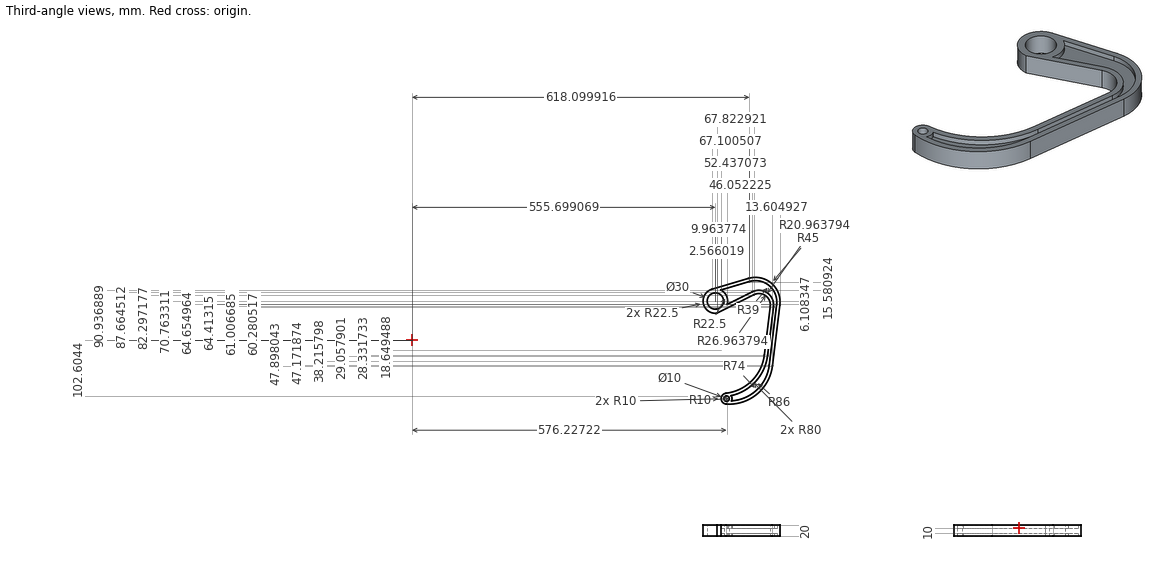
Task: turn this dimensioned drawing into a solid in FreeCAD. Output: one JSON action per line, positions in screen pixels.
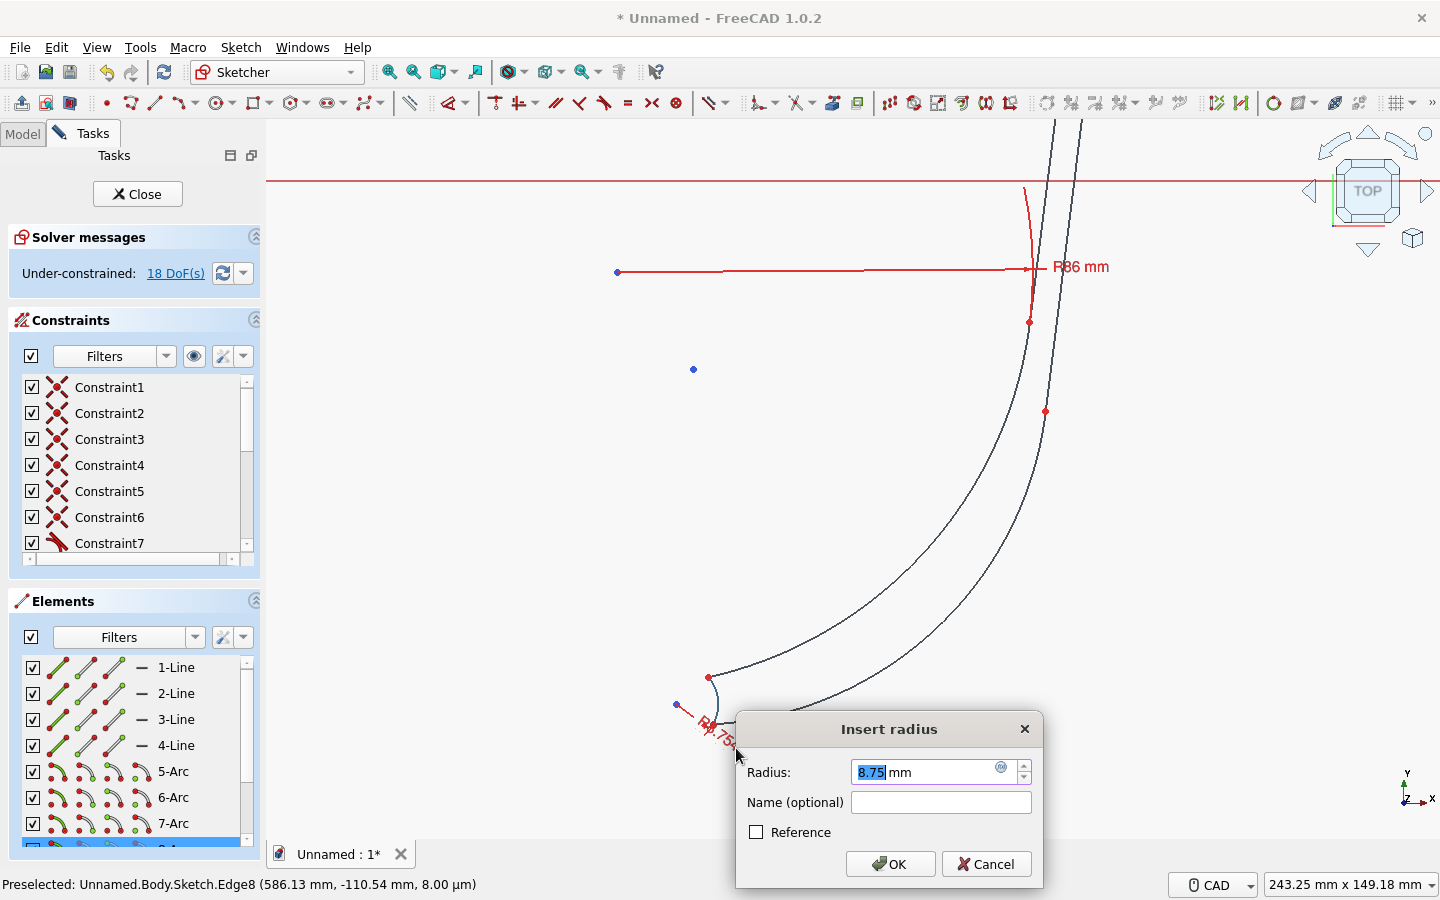
{"action": "type", "text": "10"}
{"action": "key", "text": "Return"}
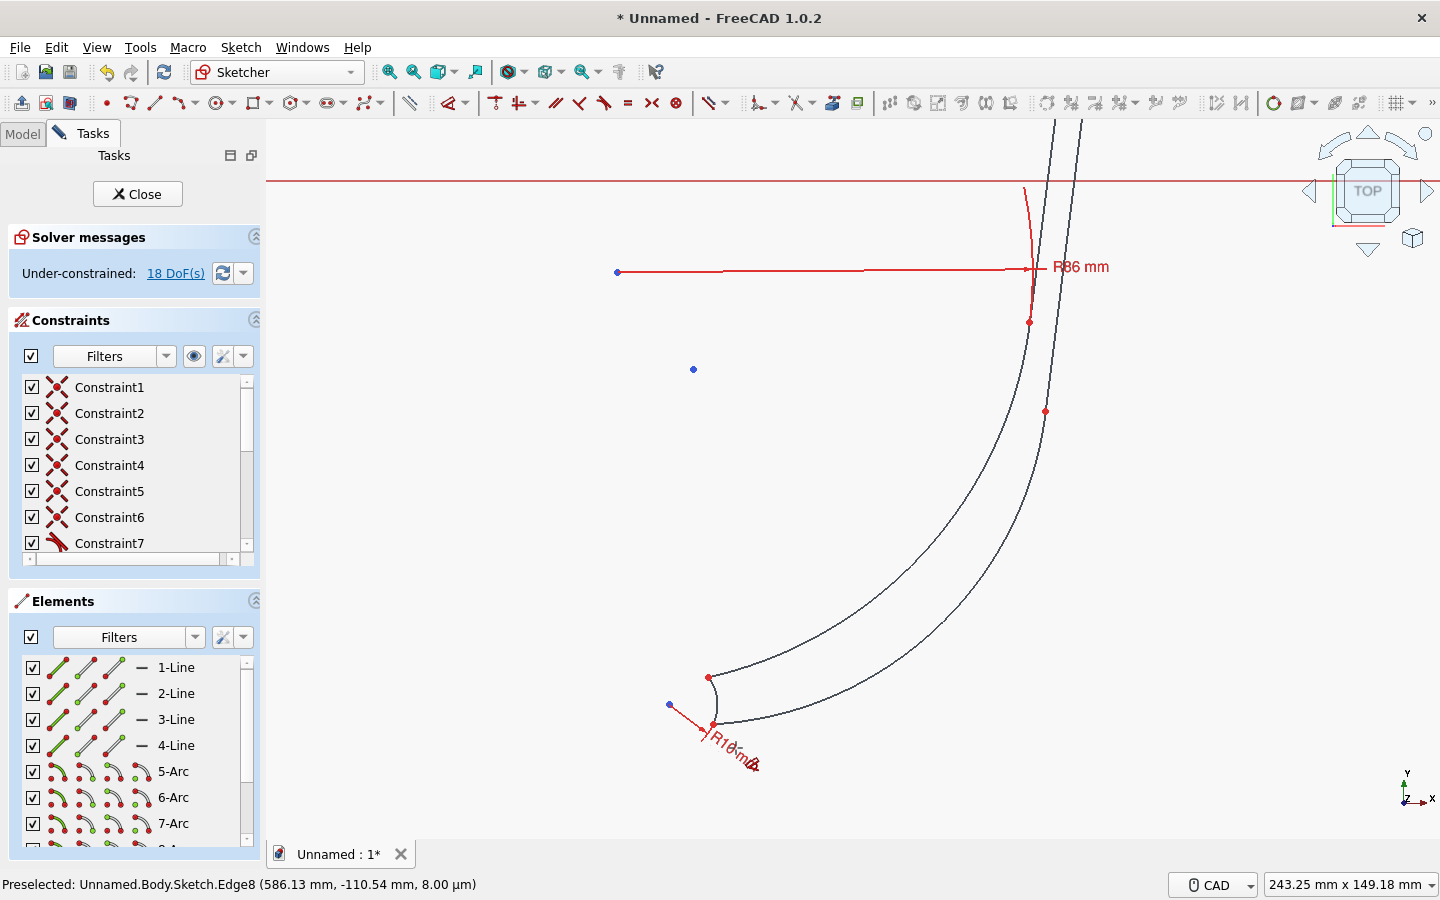
{"action": "left_click", "coordinate": [856, 685]}
{"action": "left_click", "coordinate": [871, 713]}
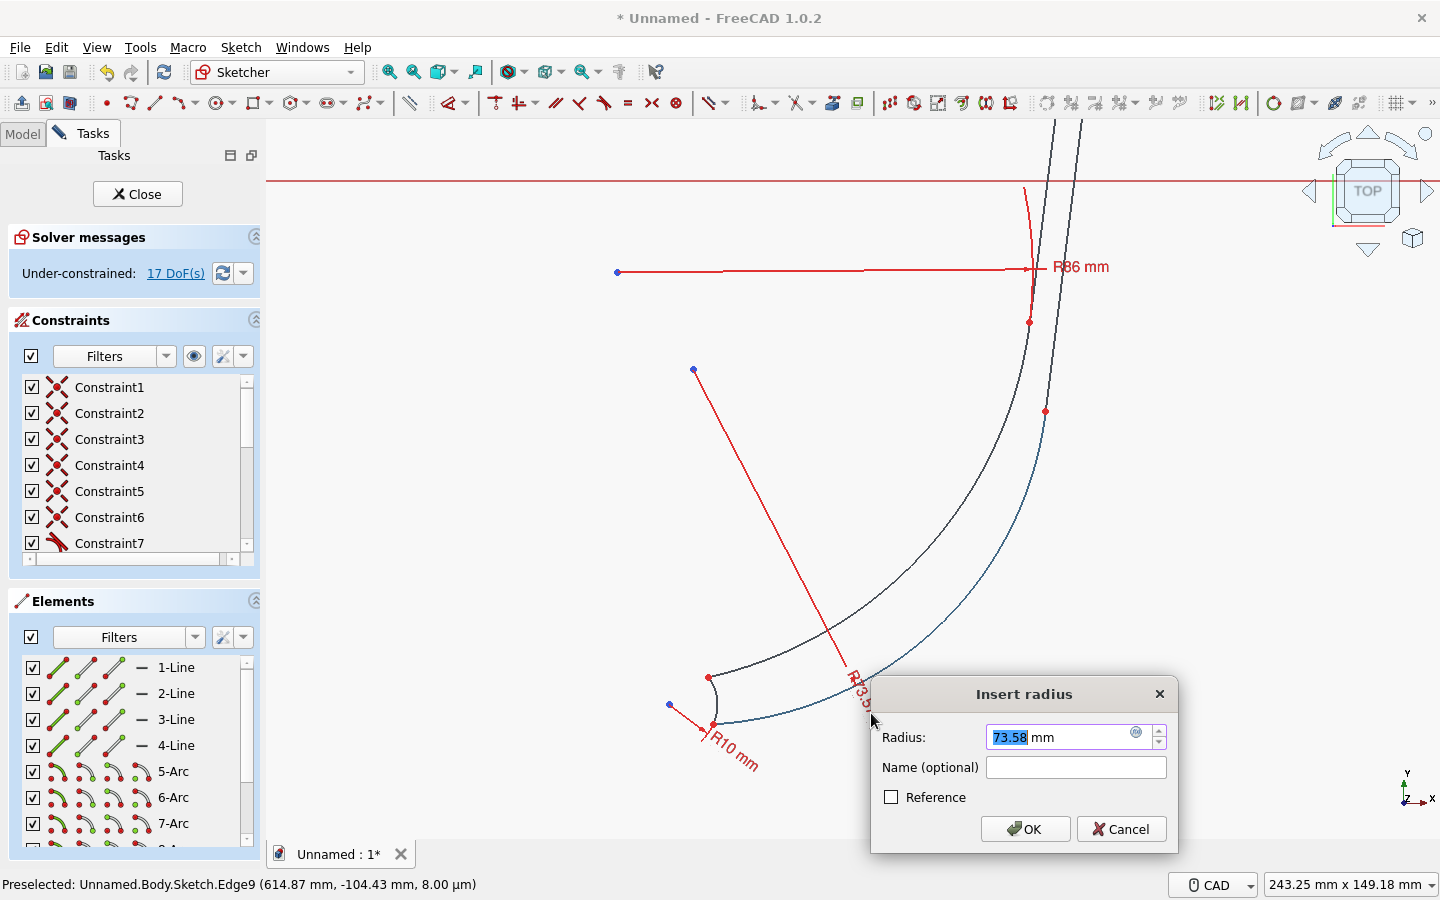
{"action": "type", "text": "74"}
{"action": "key", "text": "Return"}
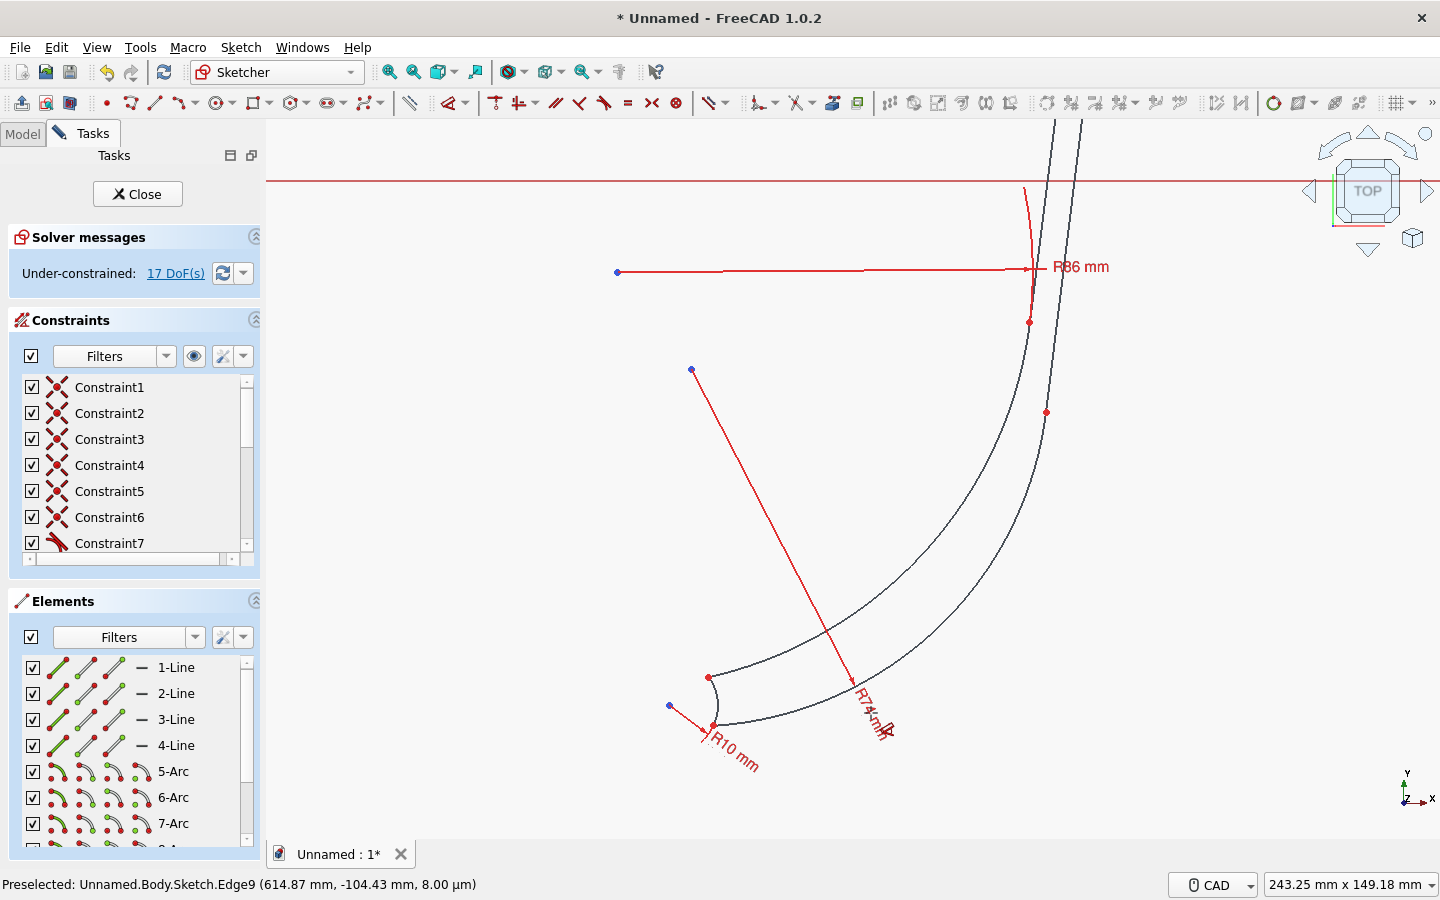
{"action": "scroll", "coordinate": [719, 711], "scroll_direction": "down", "scroll_amount": 4}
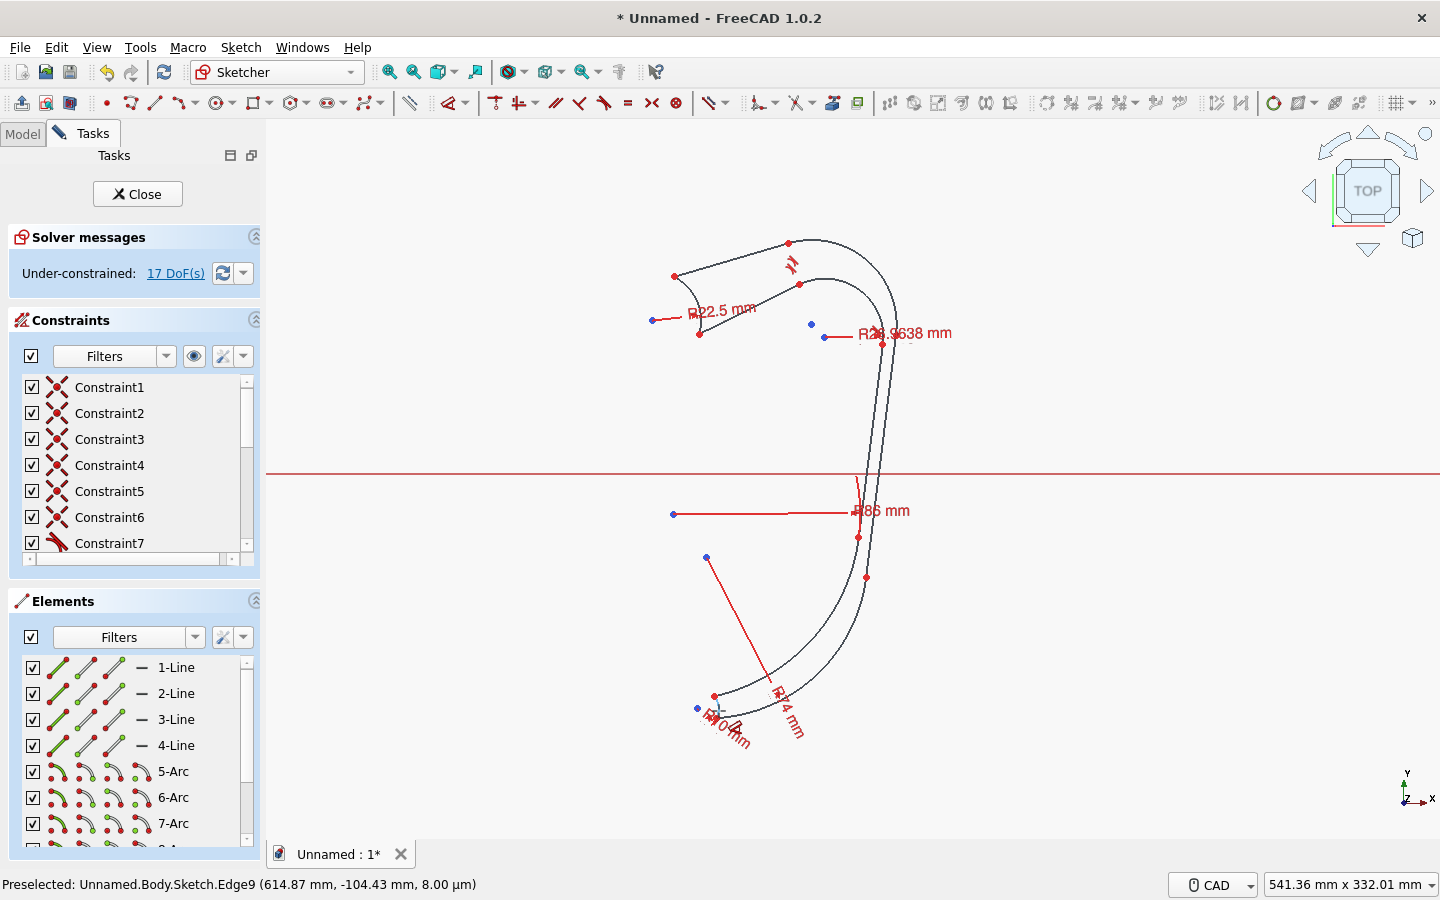
{"action": "left_click", "coordinate": [887, 286]}
{"action": "left_click", "coordinate": [915, 271]}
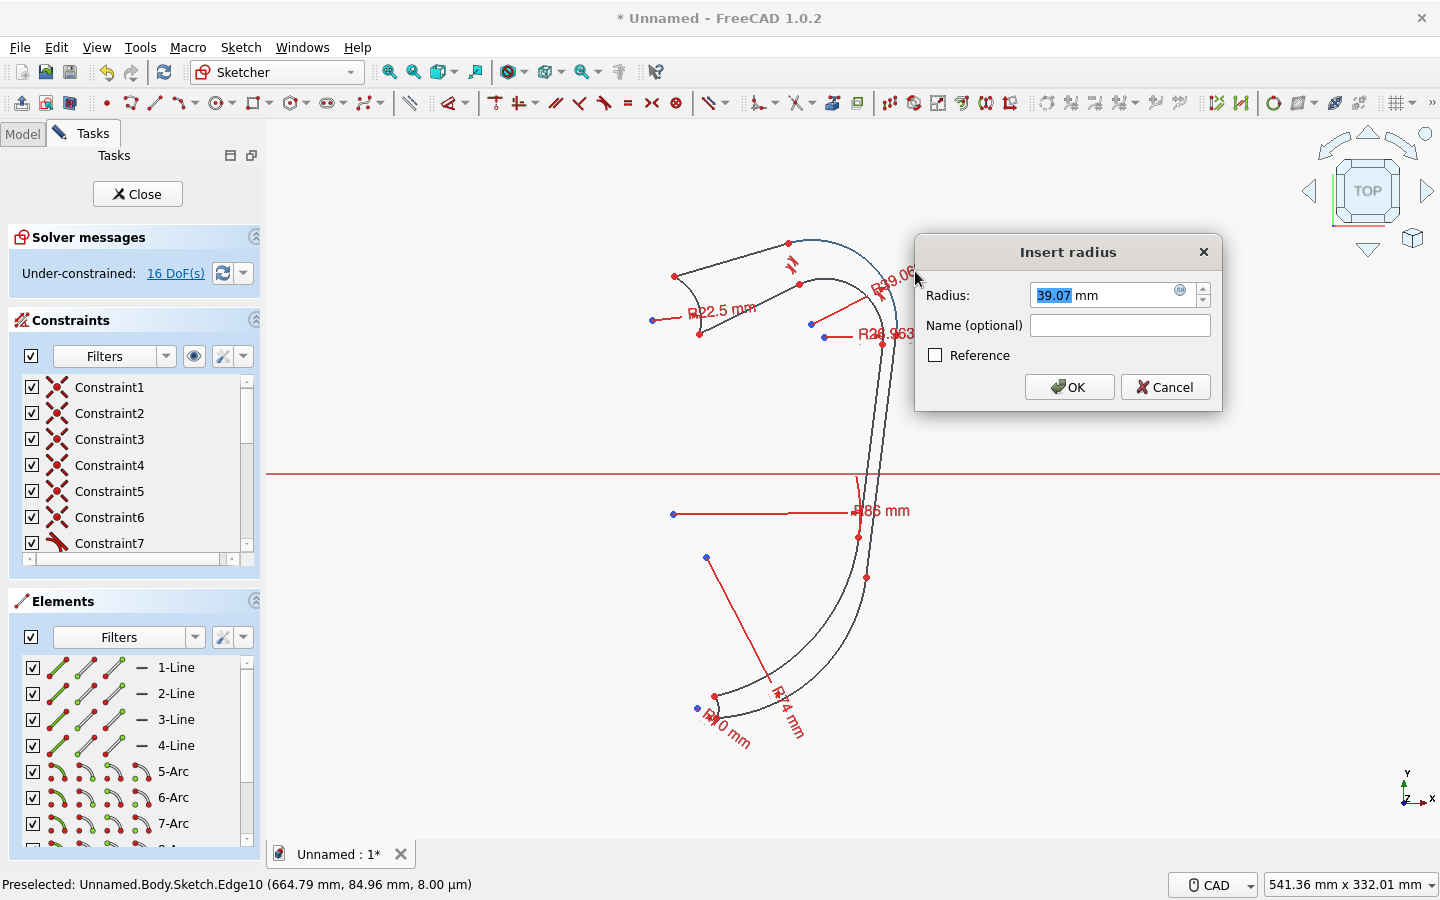
{"action": "type", "text": "39"}
{"action": "key", "text": "Return"}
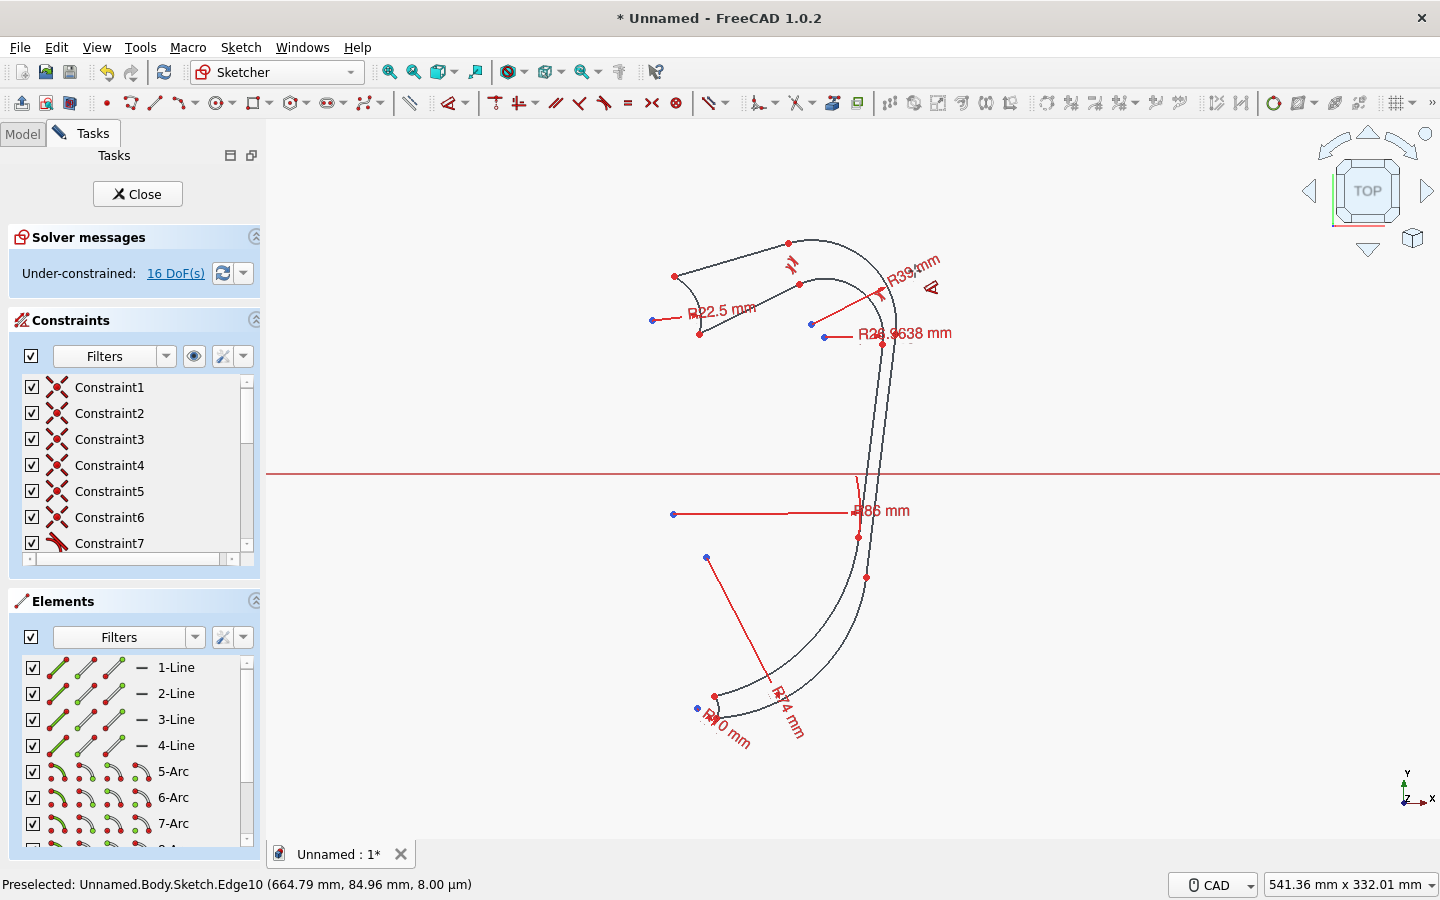
{"action": "left_click", "coordinate": [896, 335]}
{"action": "left_click", "coordinate": [930, 404]}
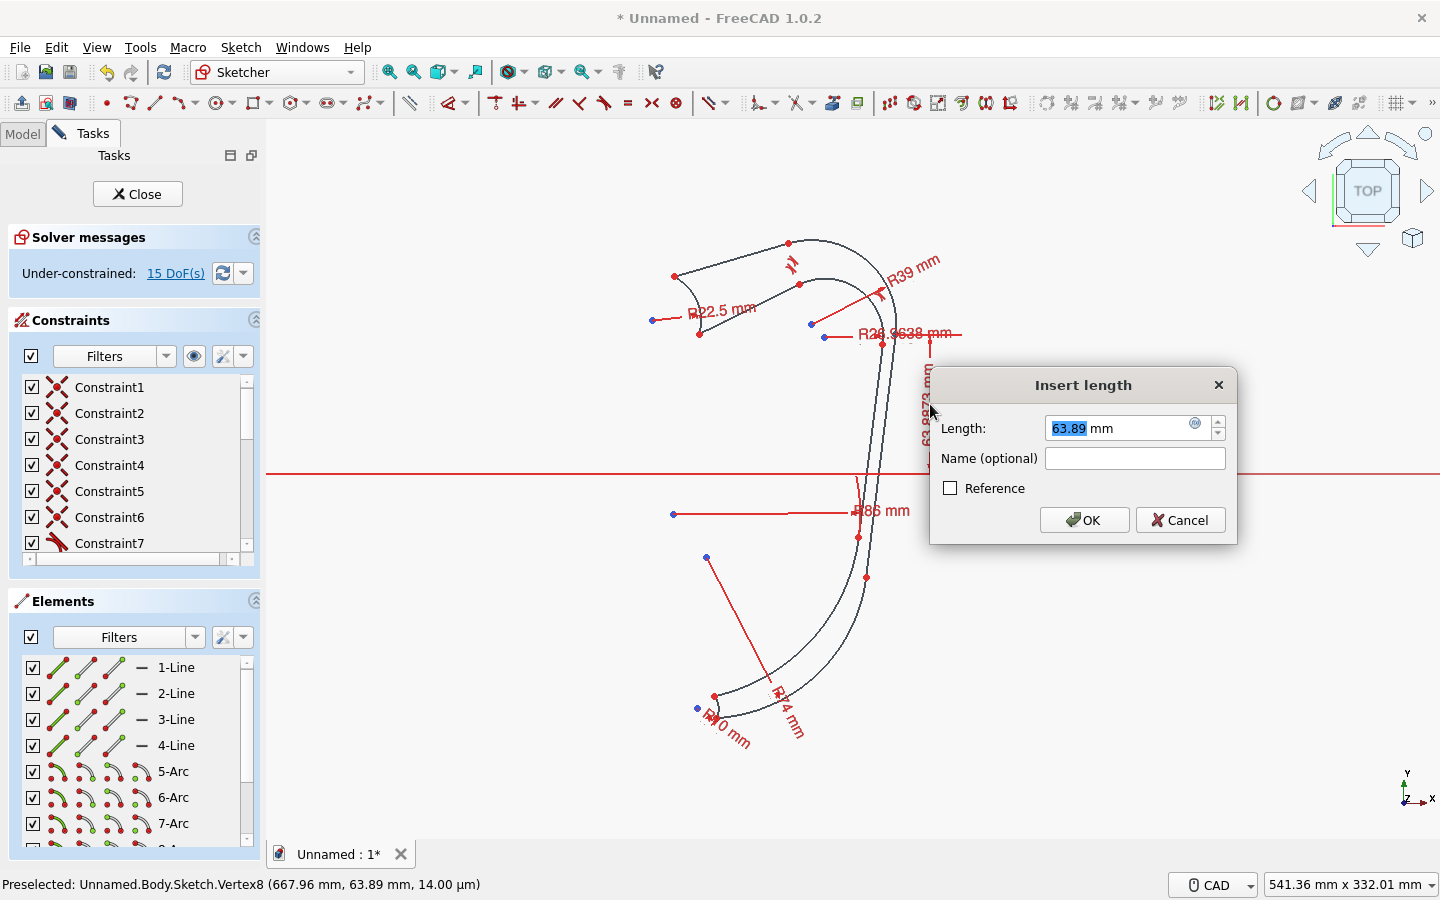
{"action": "type", "text": "64.41315"}
{"action": "key", "text": "Return"}